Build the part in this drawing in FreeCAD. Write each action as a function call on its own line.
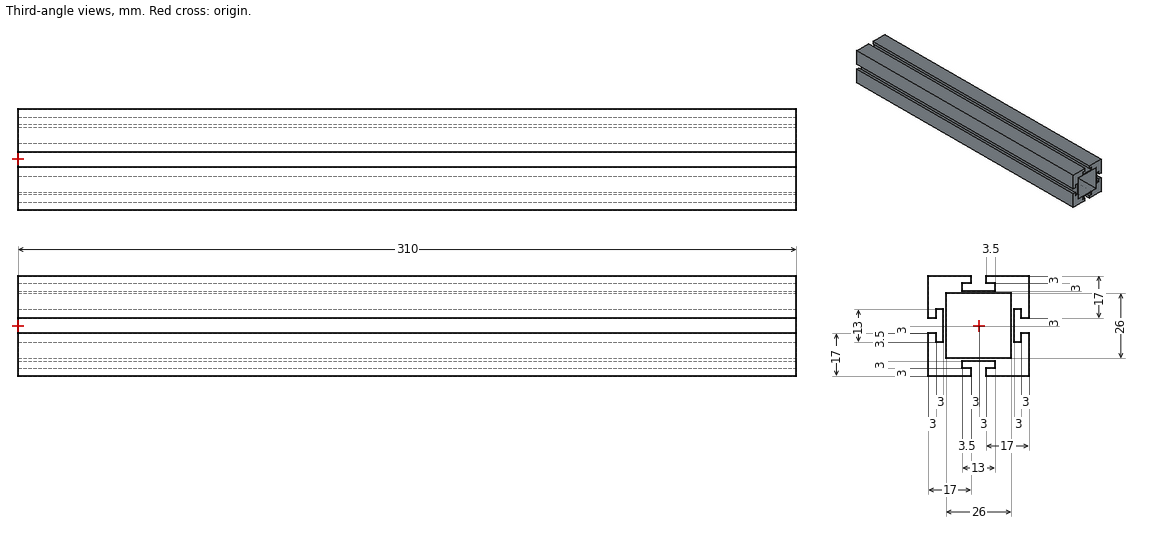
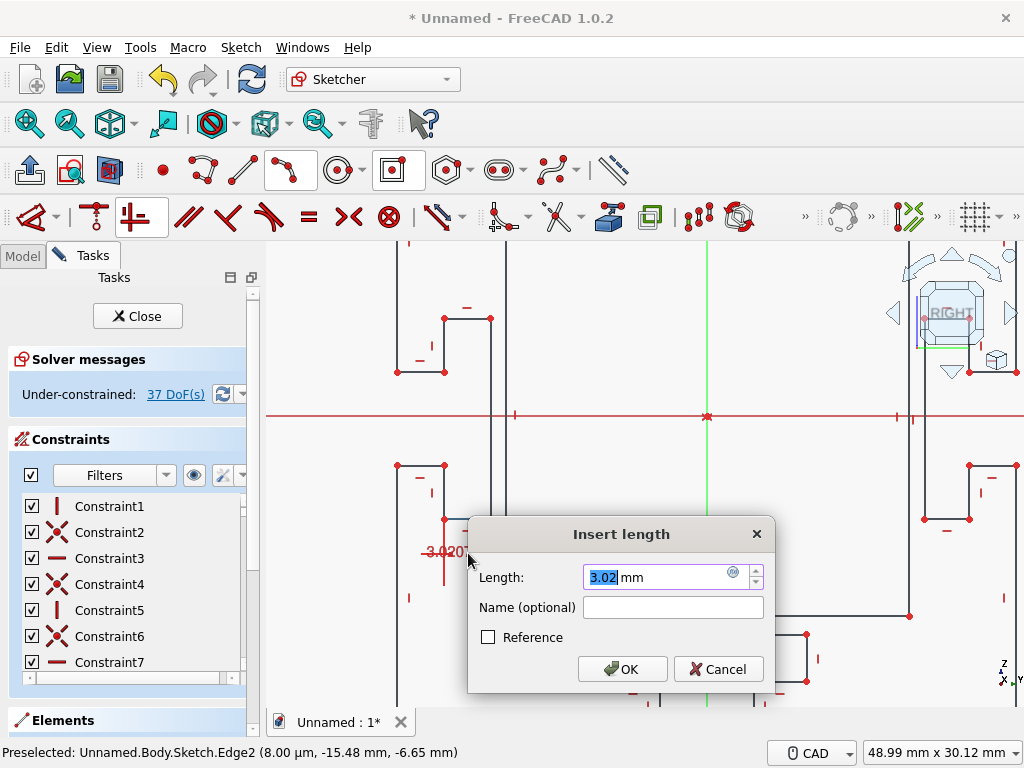
text(3)
key(Return)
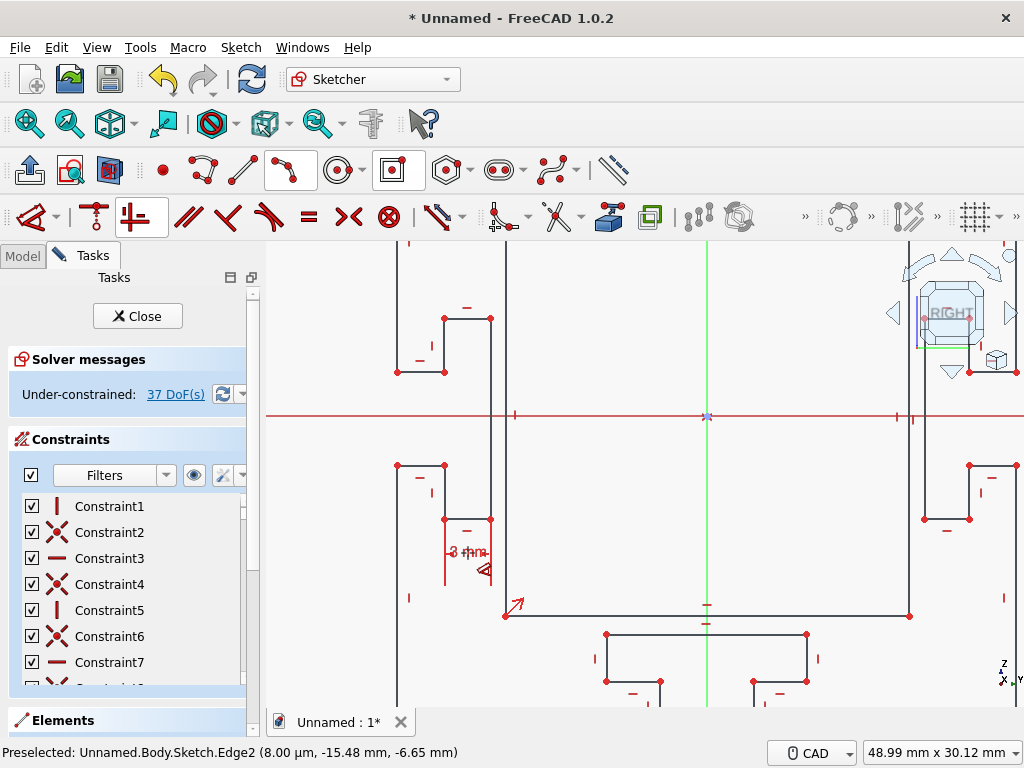
click(430, 466)
click(421, 500)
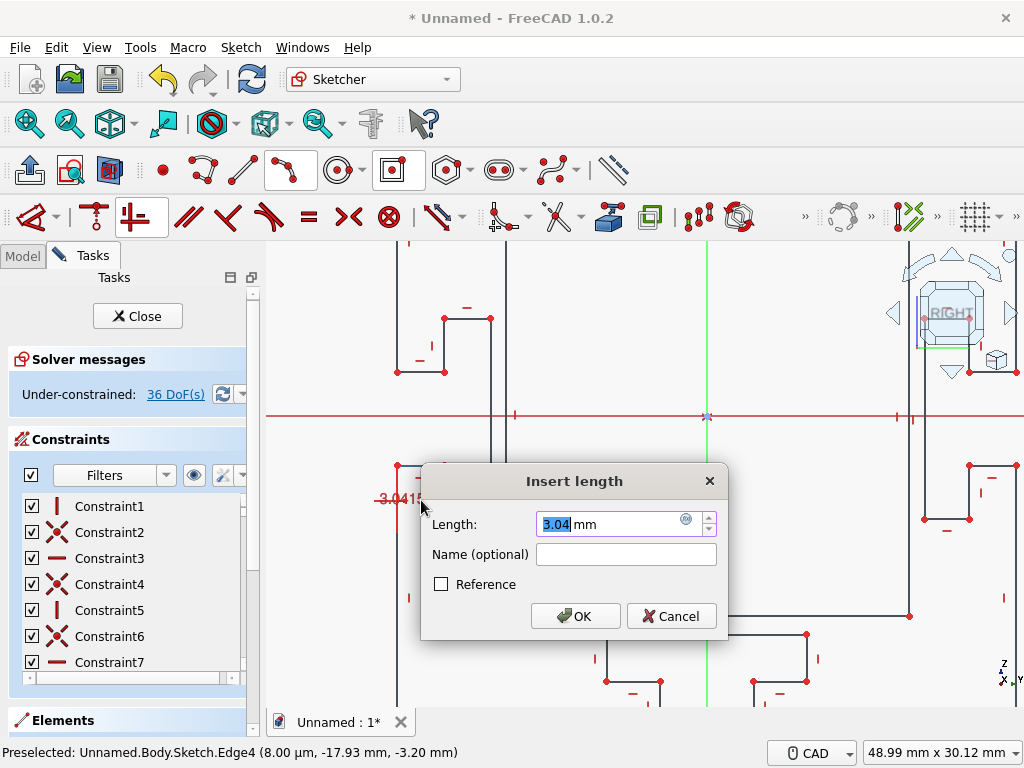
text(3)
key(Return)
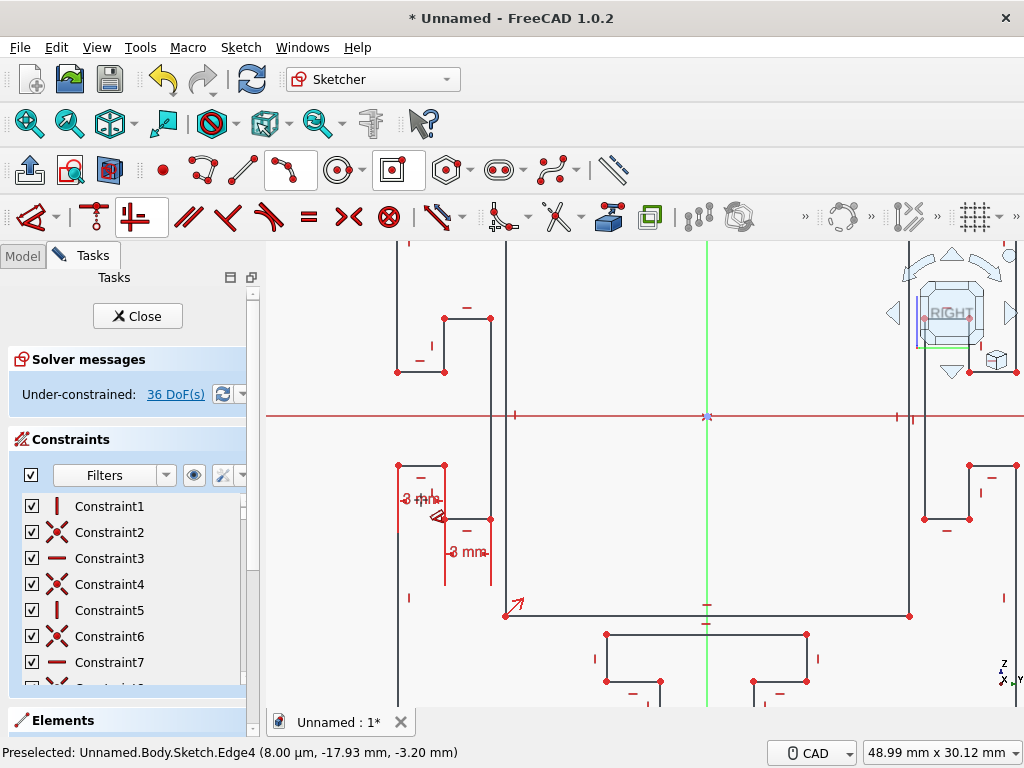
scroll(470, 521, down, 4)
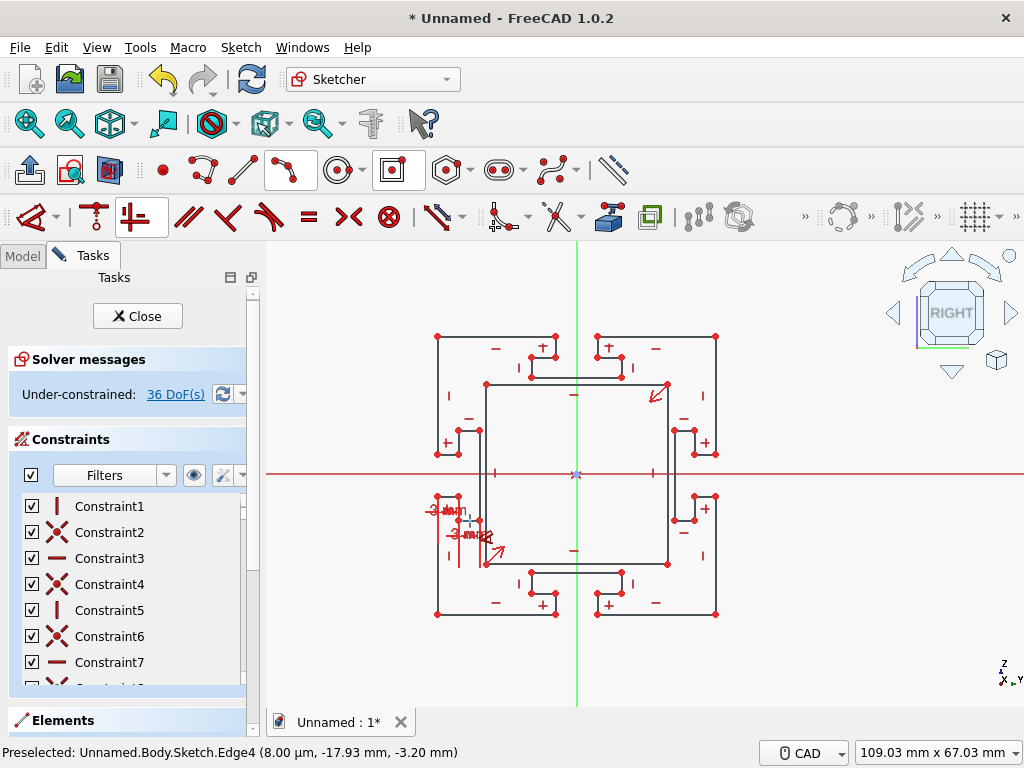
scroll(556, 608, up, 4)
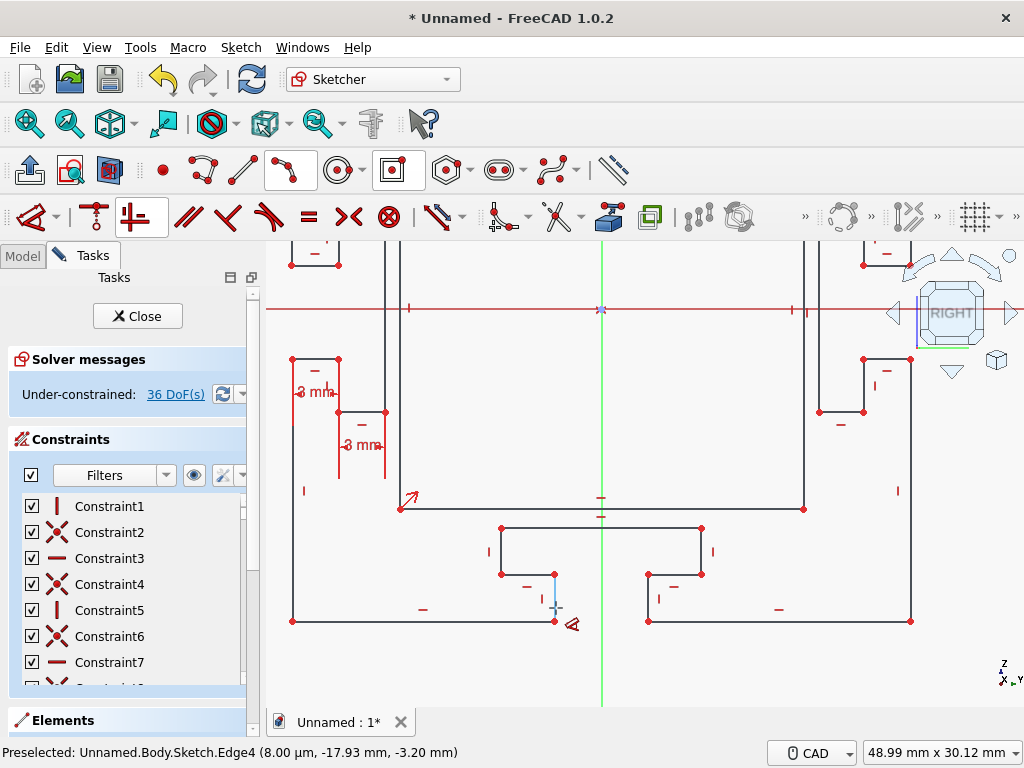
click(555, 608)
click(521, 598)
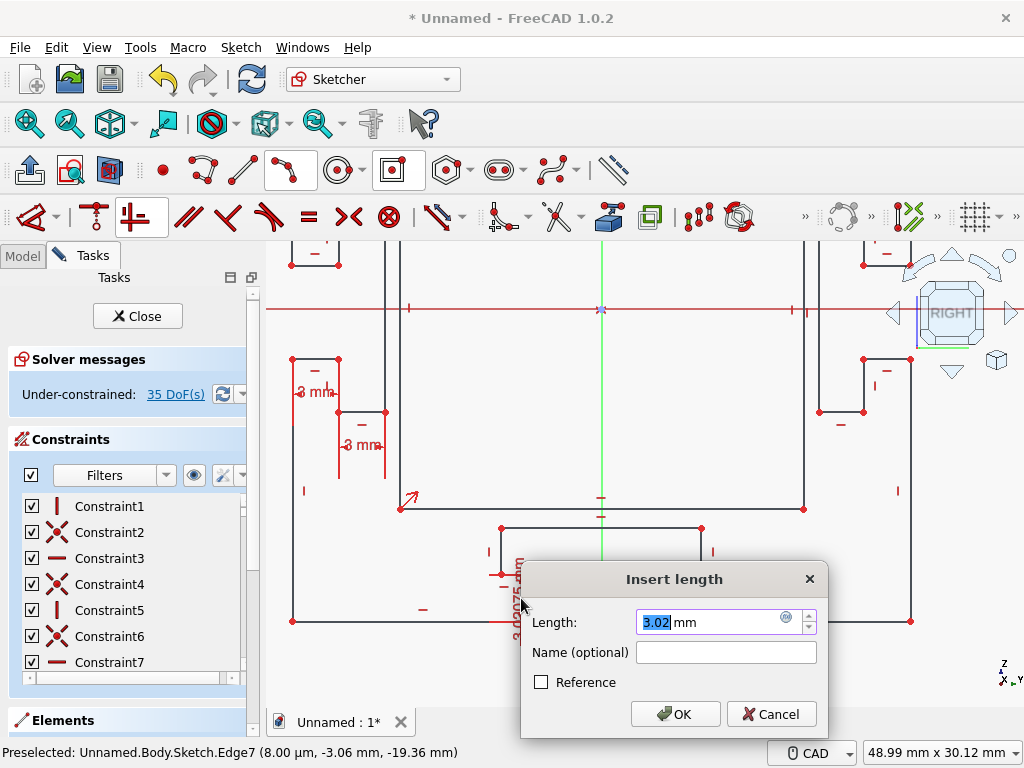
text(3)
key(Return)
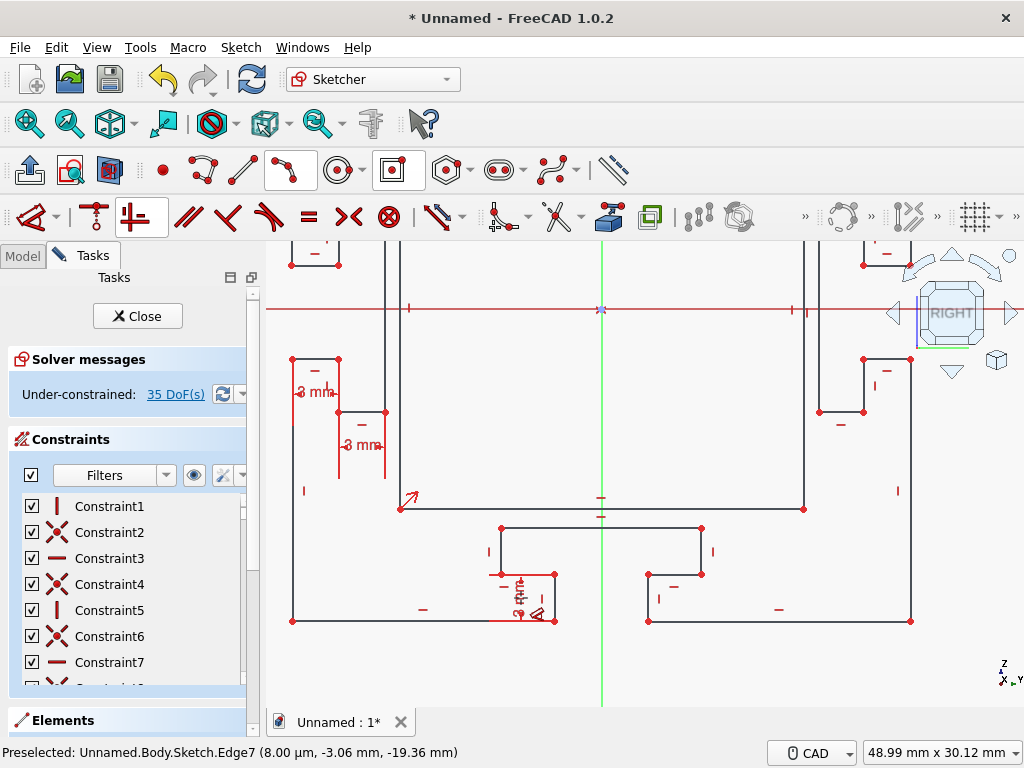
click(501, 561)
click(467, 552)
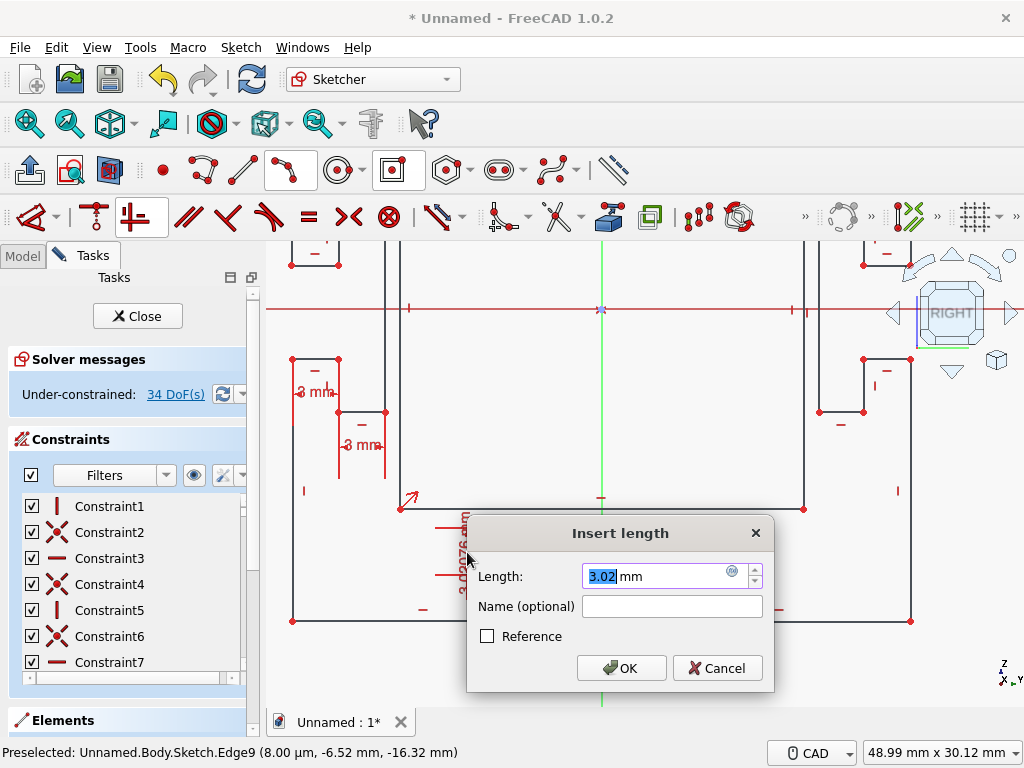
text(3)
key(Return)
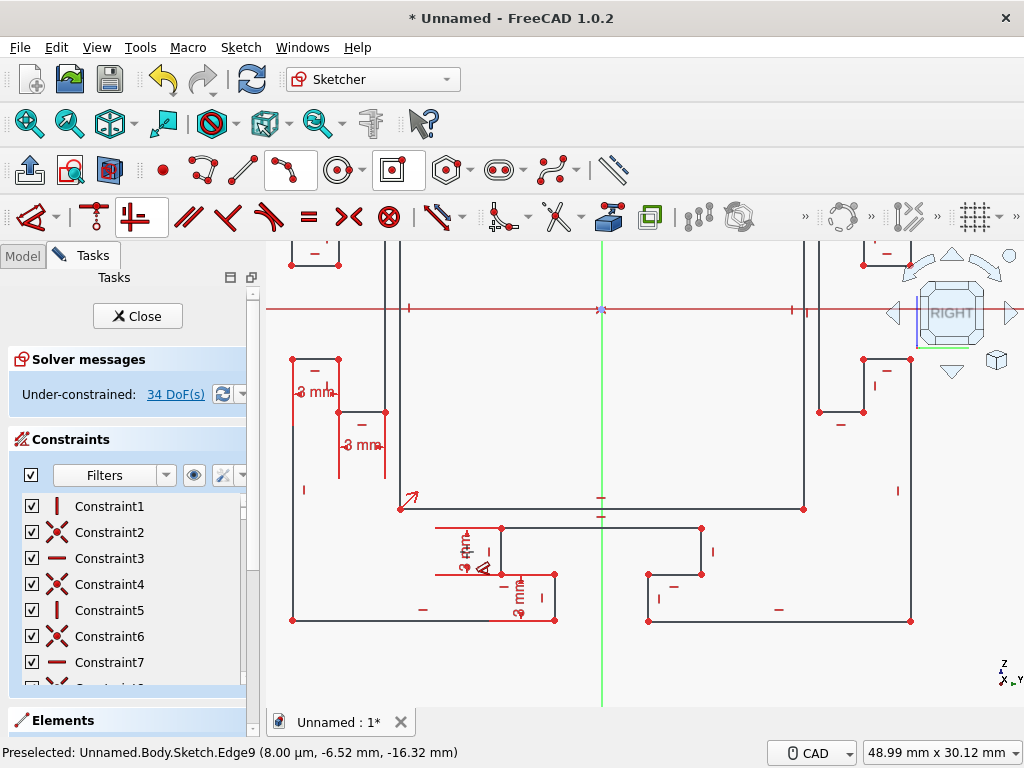
click(701, 542)
click(735, 552)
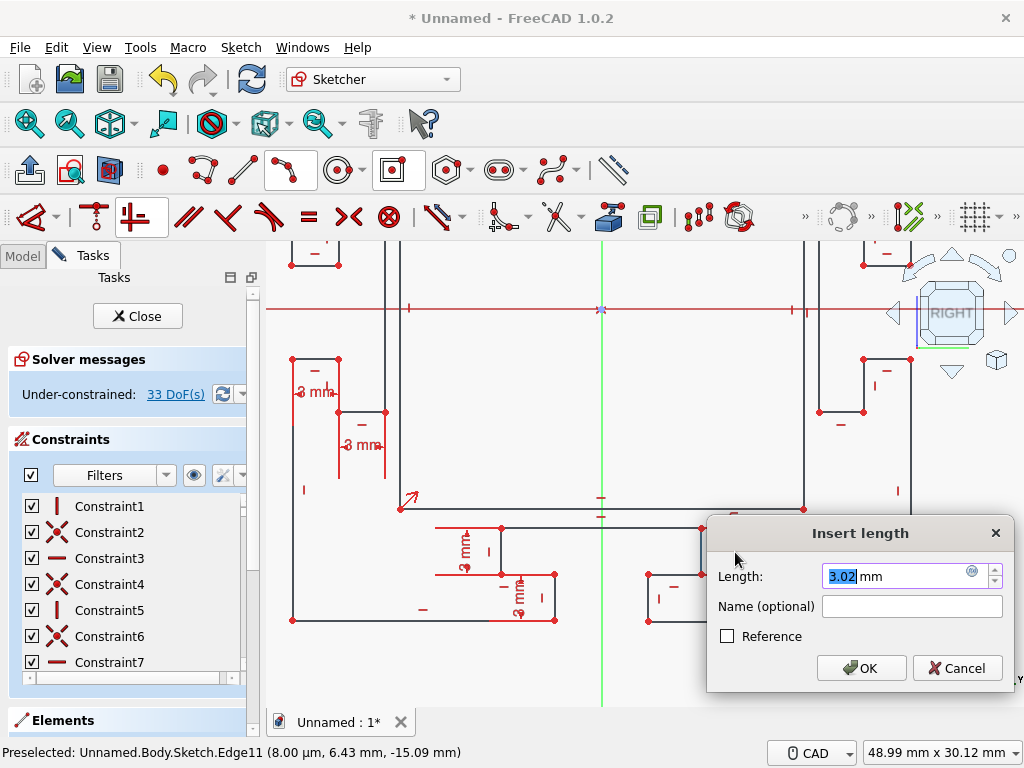
text(3)
key(Return)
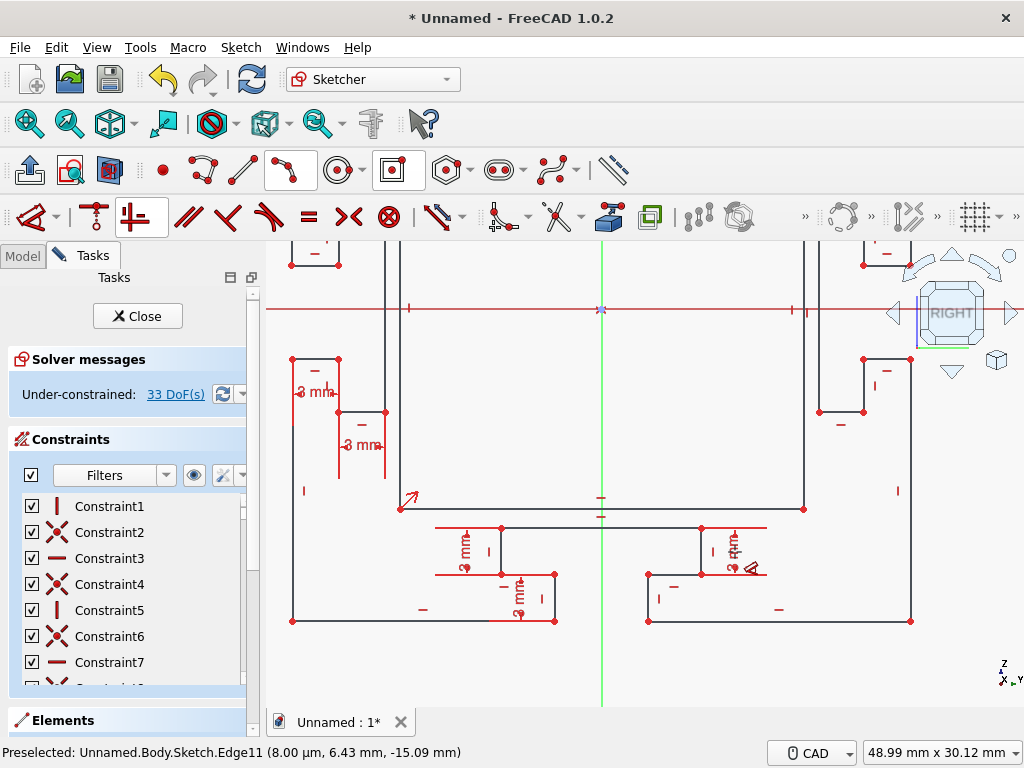
click(648, 589)
click(682, 598)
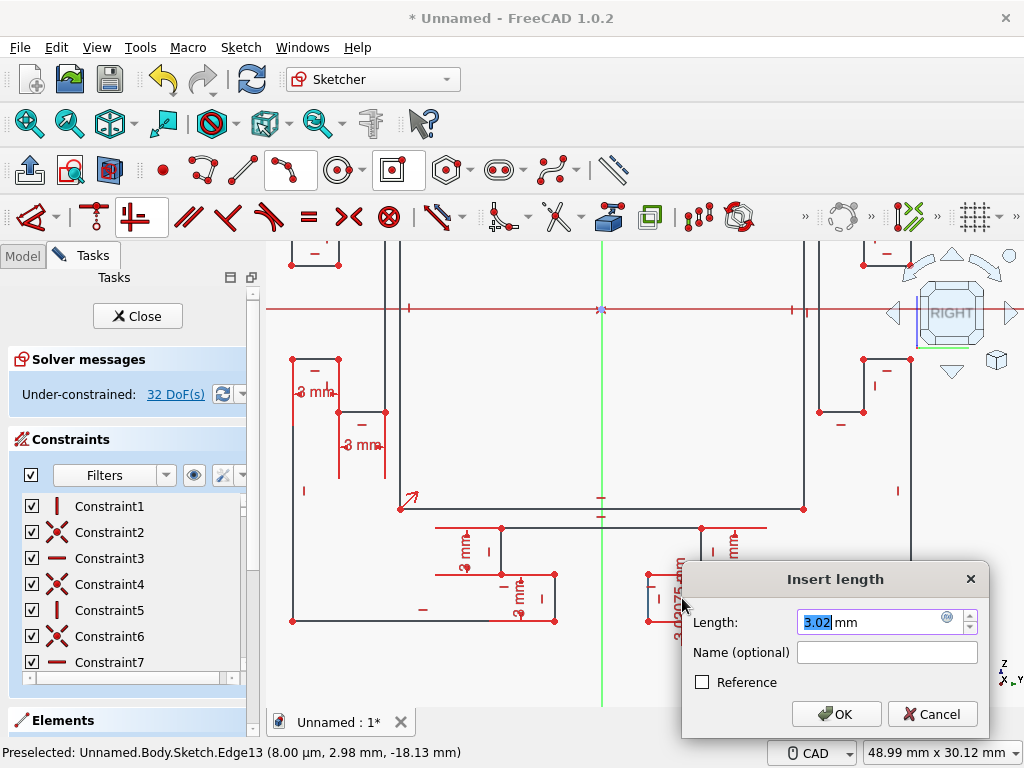
text(3)
key(Return)